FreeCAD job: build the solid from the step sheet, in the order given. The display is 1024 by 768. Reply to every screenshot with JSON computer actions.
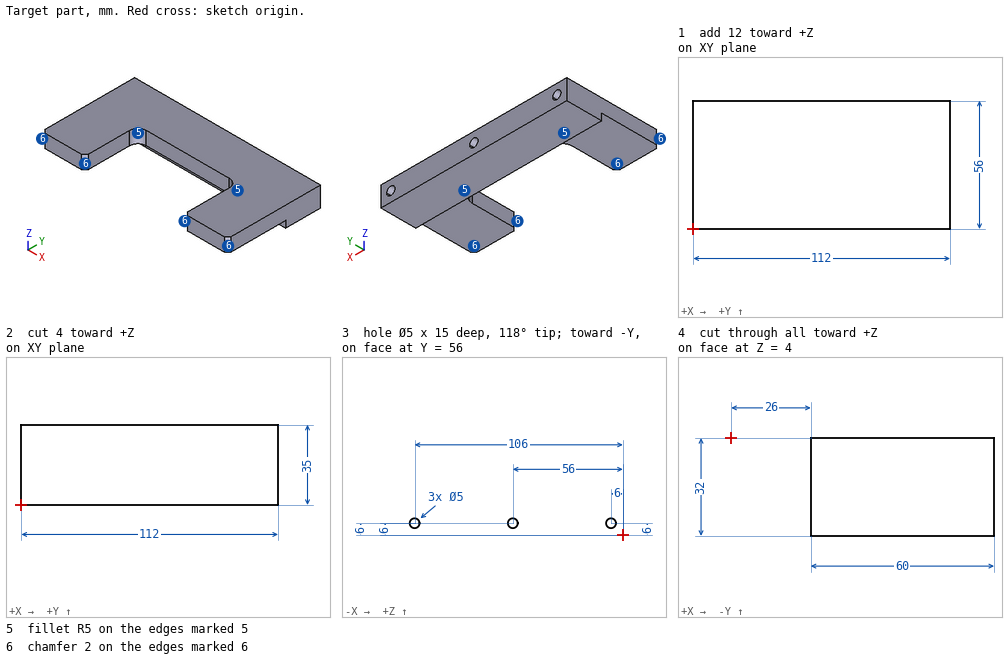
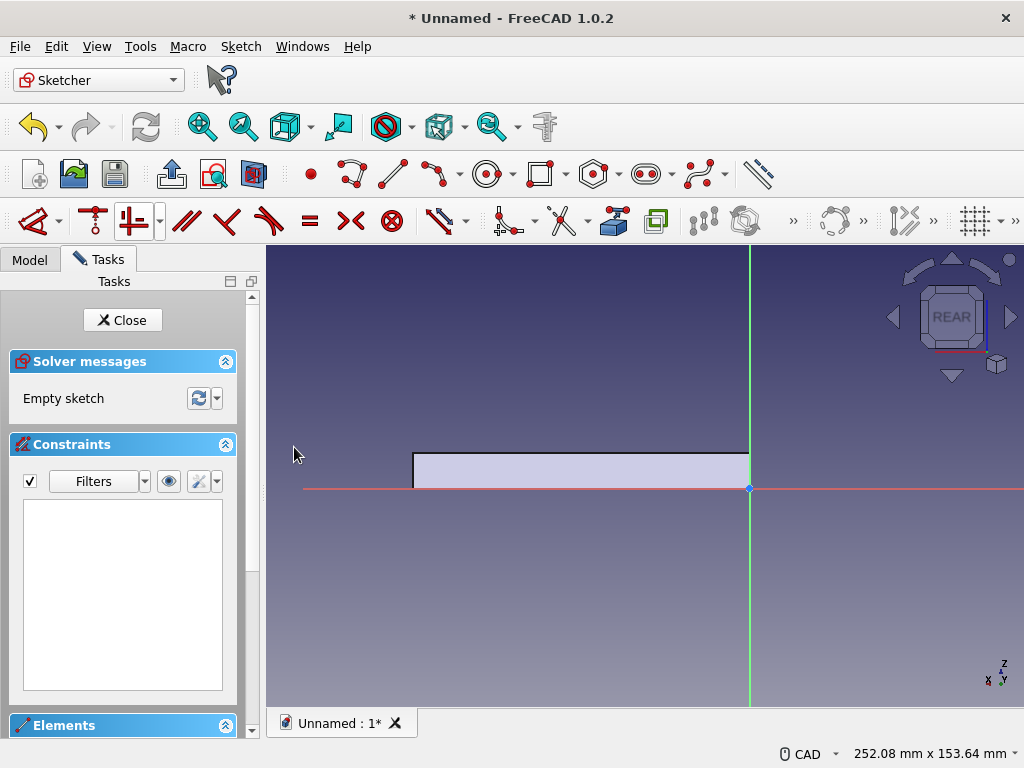
{"action": "key", "text": "g c"}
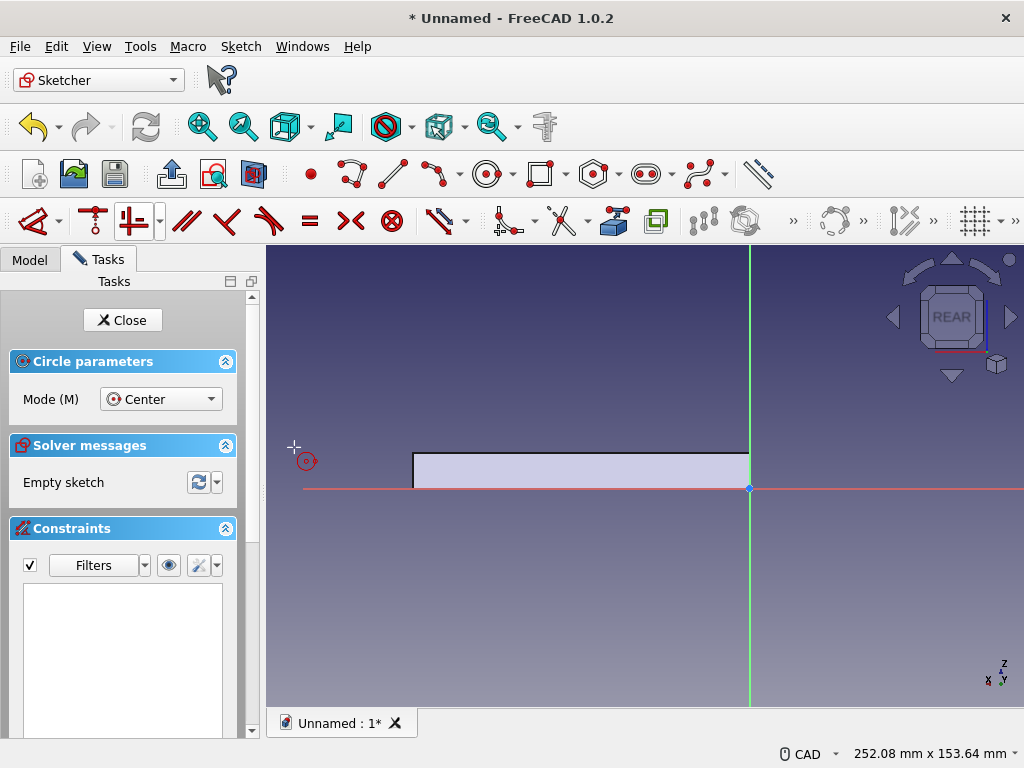
{"action": "scroll", "coordinate": [431, 471], "scroll_direction": "up", "scroll_amount": 6}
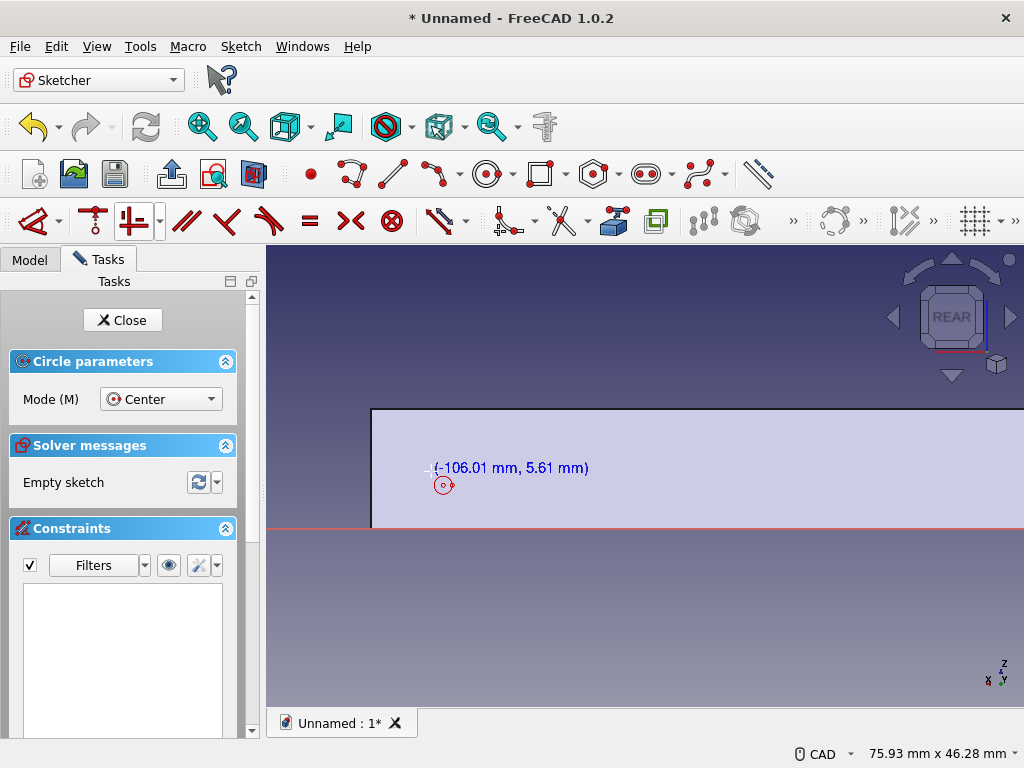
{"action": "left_click", "coordinate": [431, 469]}
{"action": "left_click", "coordinate": [448, 452]}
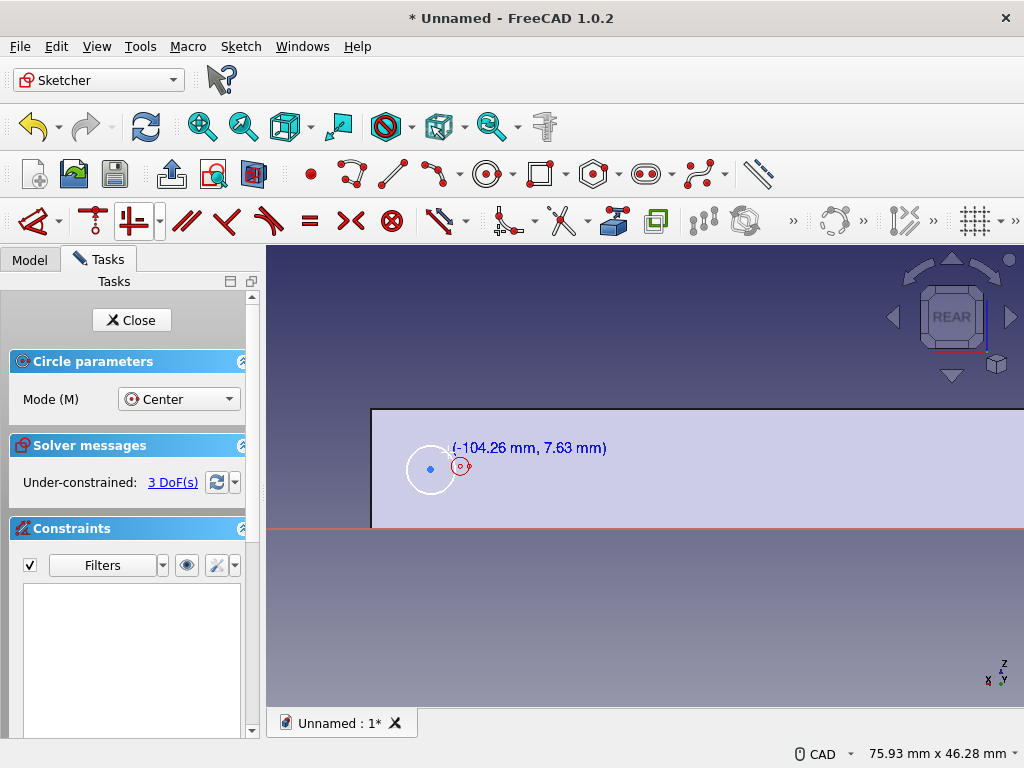
{"action": "scroll", "coordinate": [361, 470], "scroll_direction": "down", "scroll_amount": 5}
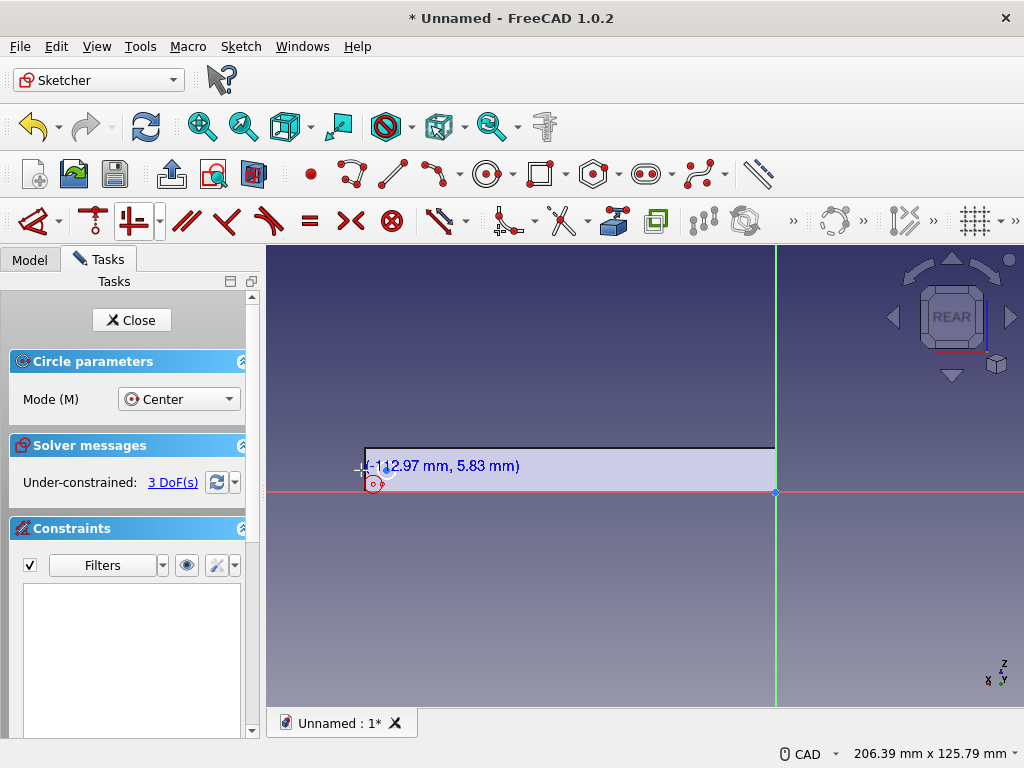
{"action": "scroll", "coordinate": [754, 470], "scroll_direction": "up", "scroll_amount": 5}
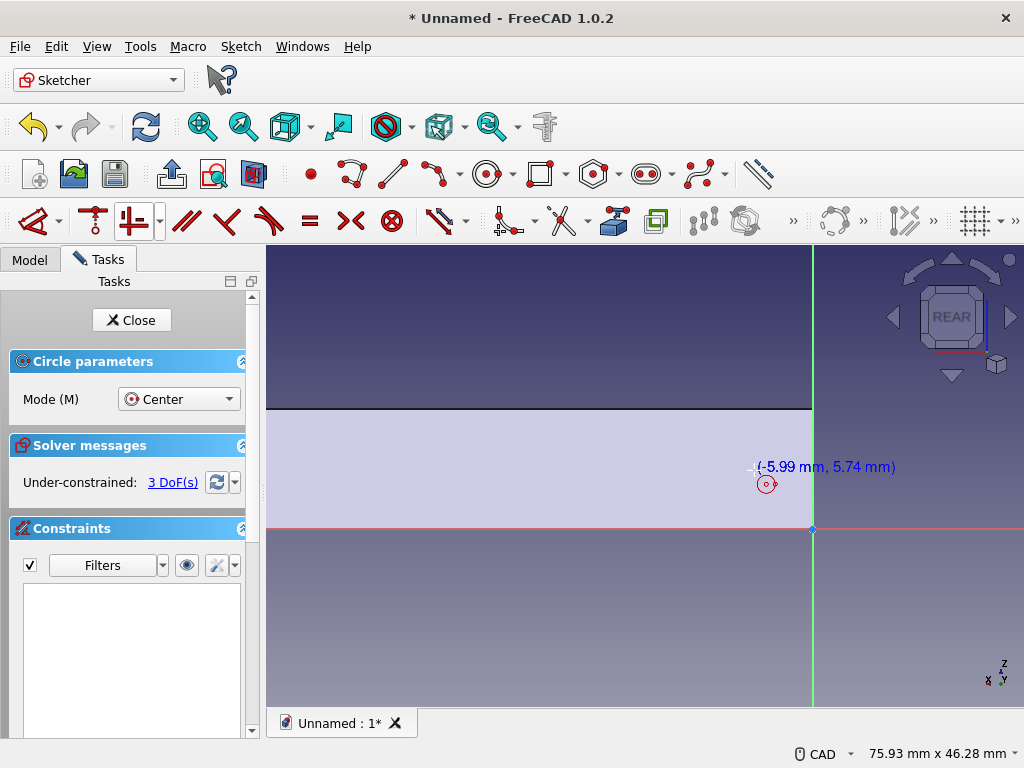
{"action": "left_click", "coordinate": [753, 469]}
{"action": "left_click", "coordinate": [770, 452]}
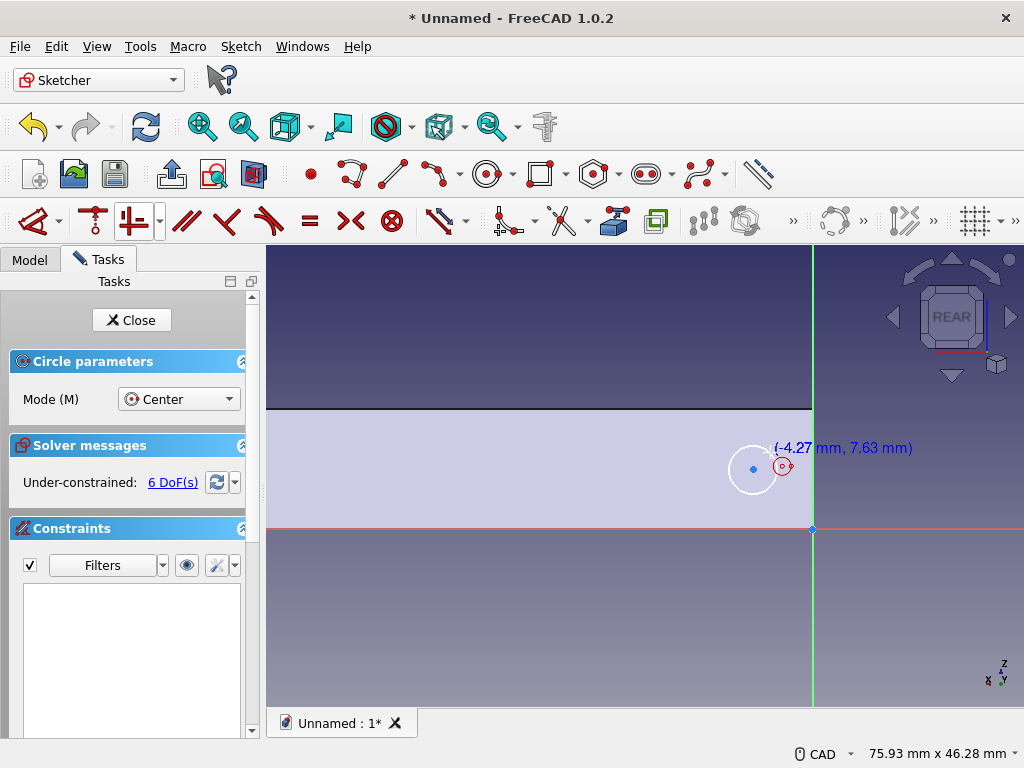
{"action": "scroll", "coordinate": [754, 470], "scroll_direction": "down", "scroll_amount": 5}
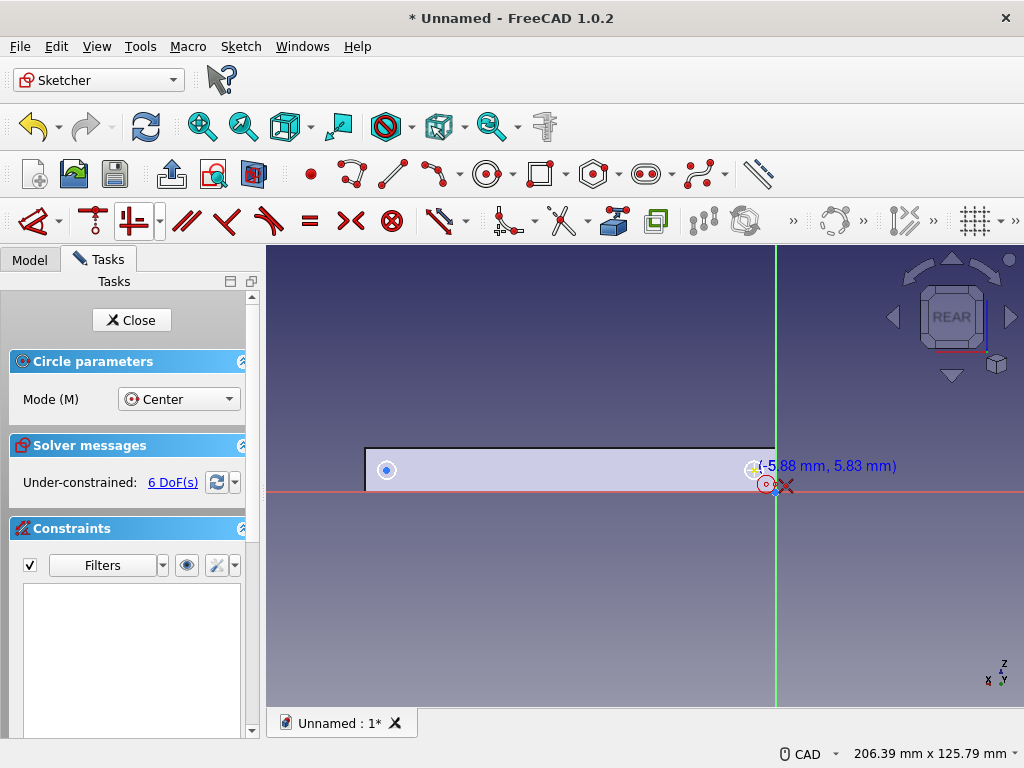
{"action": "scroll", "coordinate": [570, 470], "scroll_direction": "up", "scroll_amount": 5}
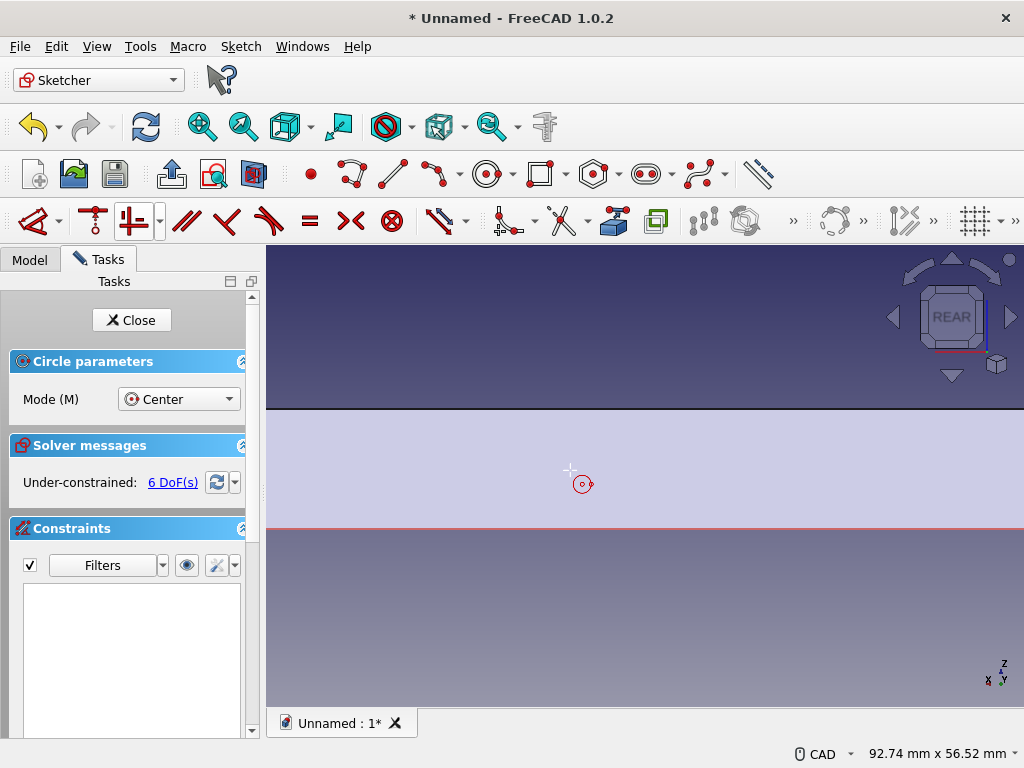
{"action": "left_click", "coordinate": [570, 469]}
{"action": "left_click", "coordinate": [588, 452]}
{"action": "key", "text": "Escape"}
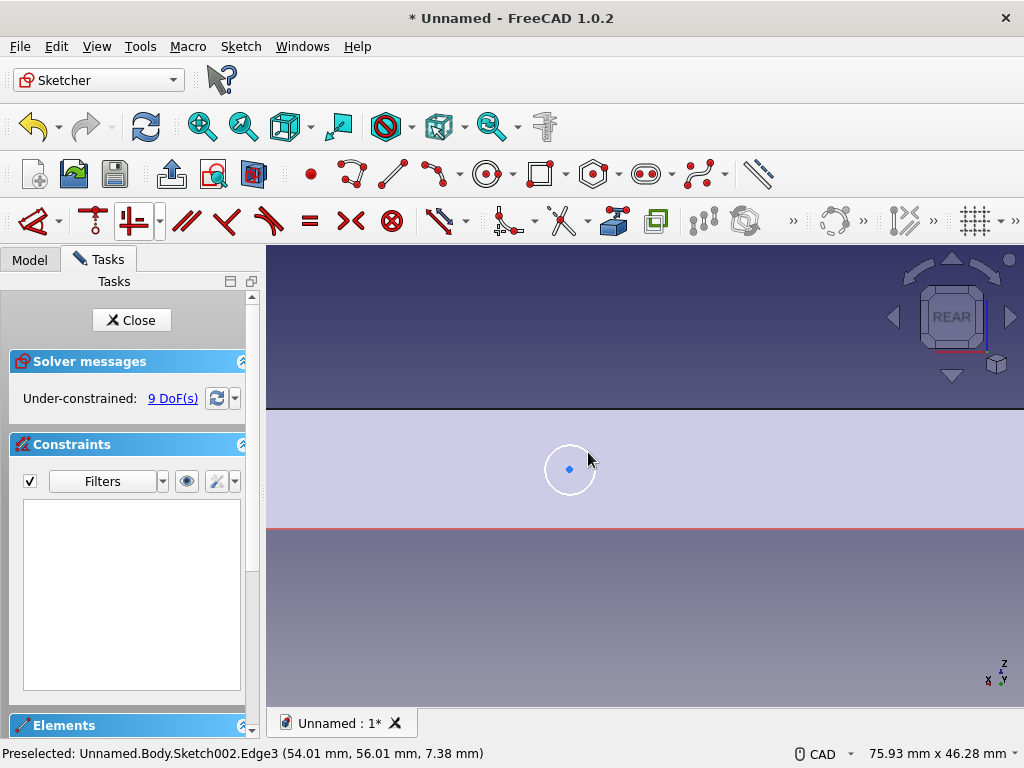
{"action": "scroll", "coordinate": [570, 470], "scroll_direction": "down", "scroll_amount": 5}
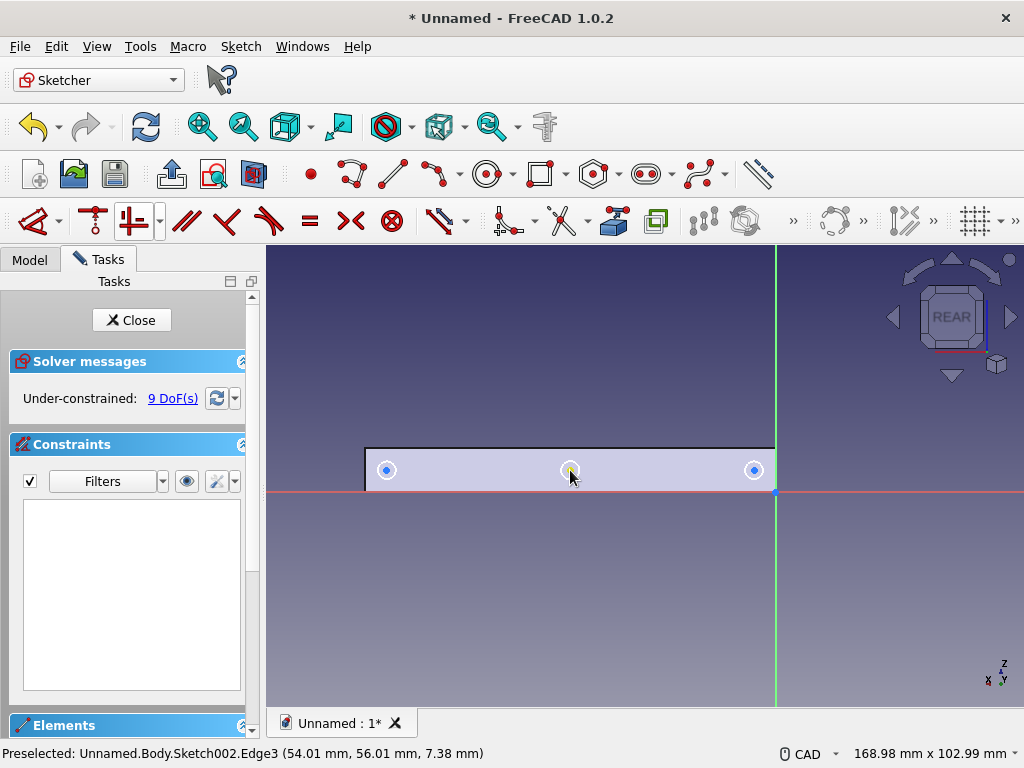
{"action": "scroll", "coordinate": [393, 464], "scroll_direction": "up", "scroll_amount": 3}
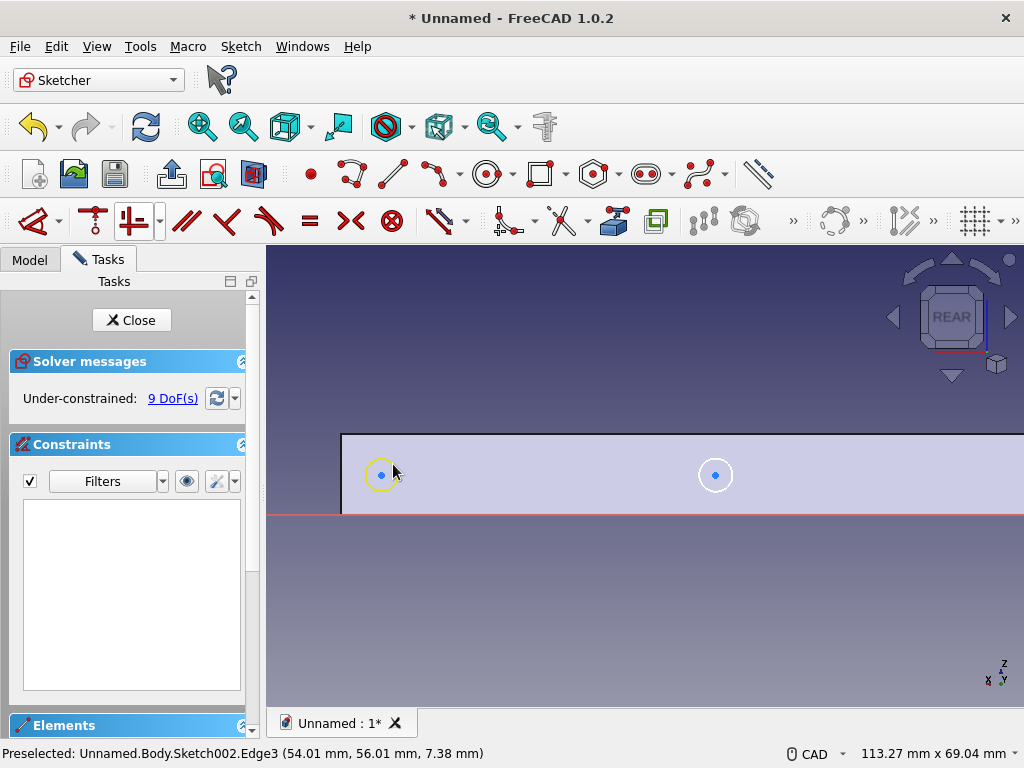
{"action": "left_click", "coordinate": [393, 464]}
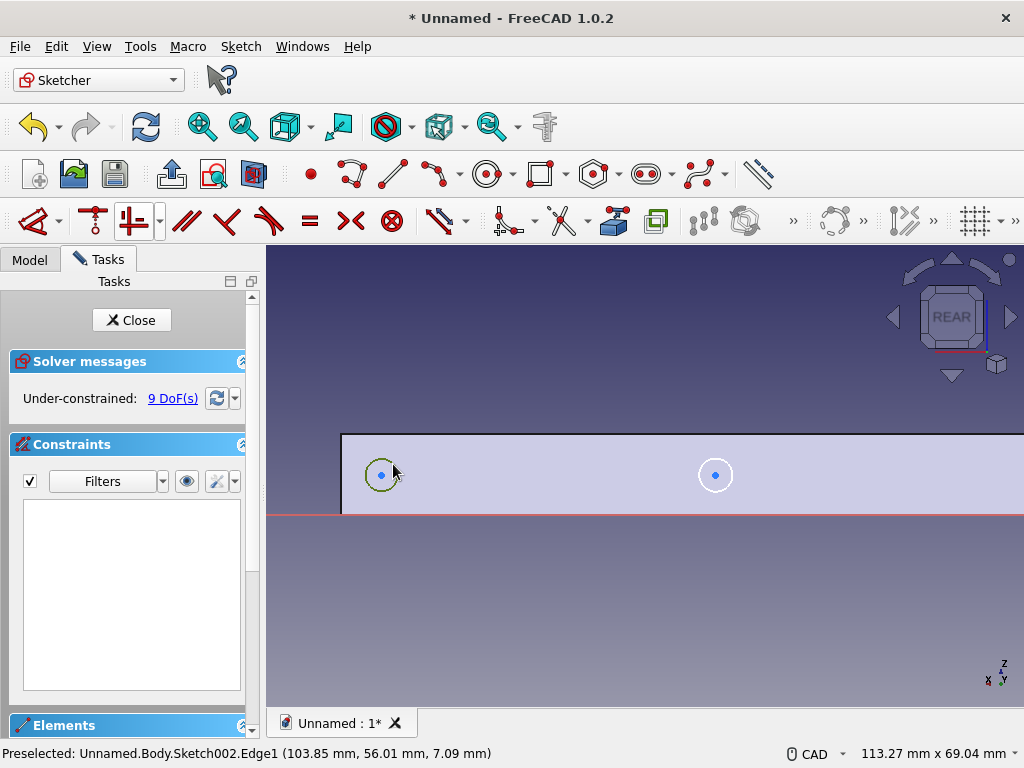
{"action": "scroll", "coordinate": [393, 463], "scroll_direction": "down", "scroll_amount": 3}